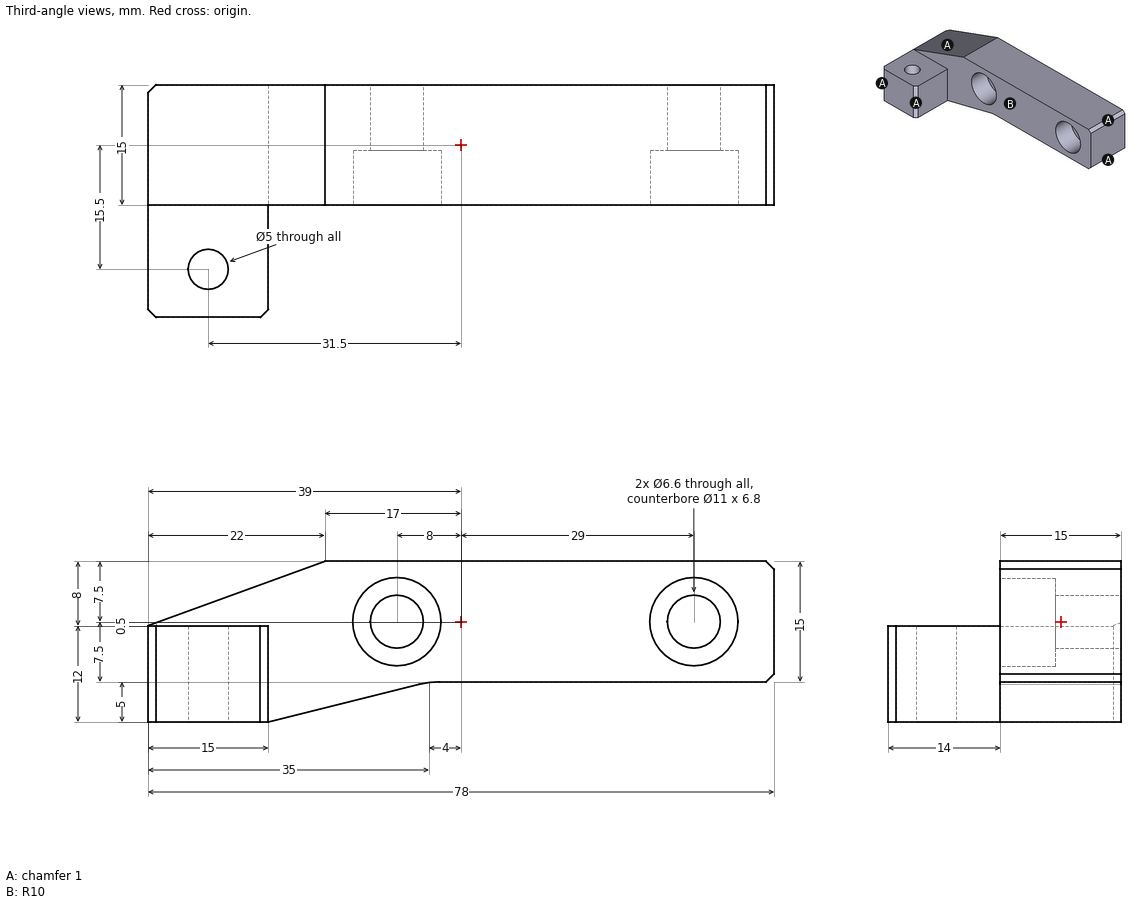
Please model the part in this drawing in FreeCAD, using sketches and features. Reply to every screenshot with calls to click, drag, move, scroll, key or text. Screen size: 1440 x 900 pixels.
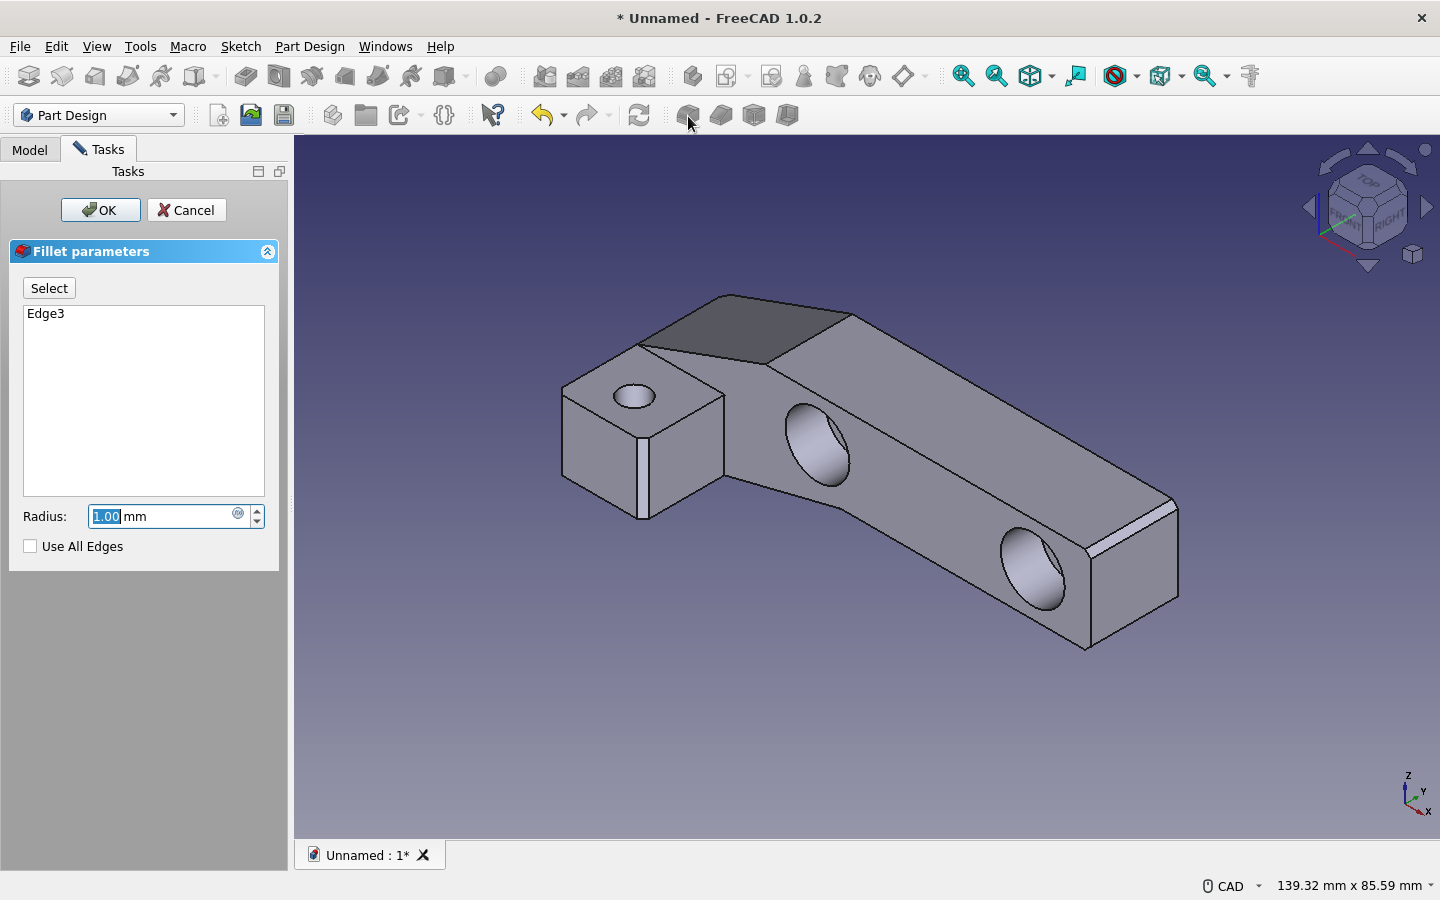
text(10)
key(Tab)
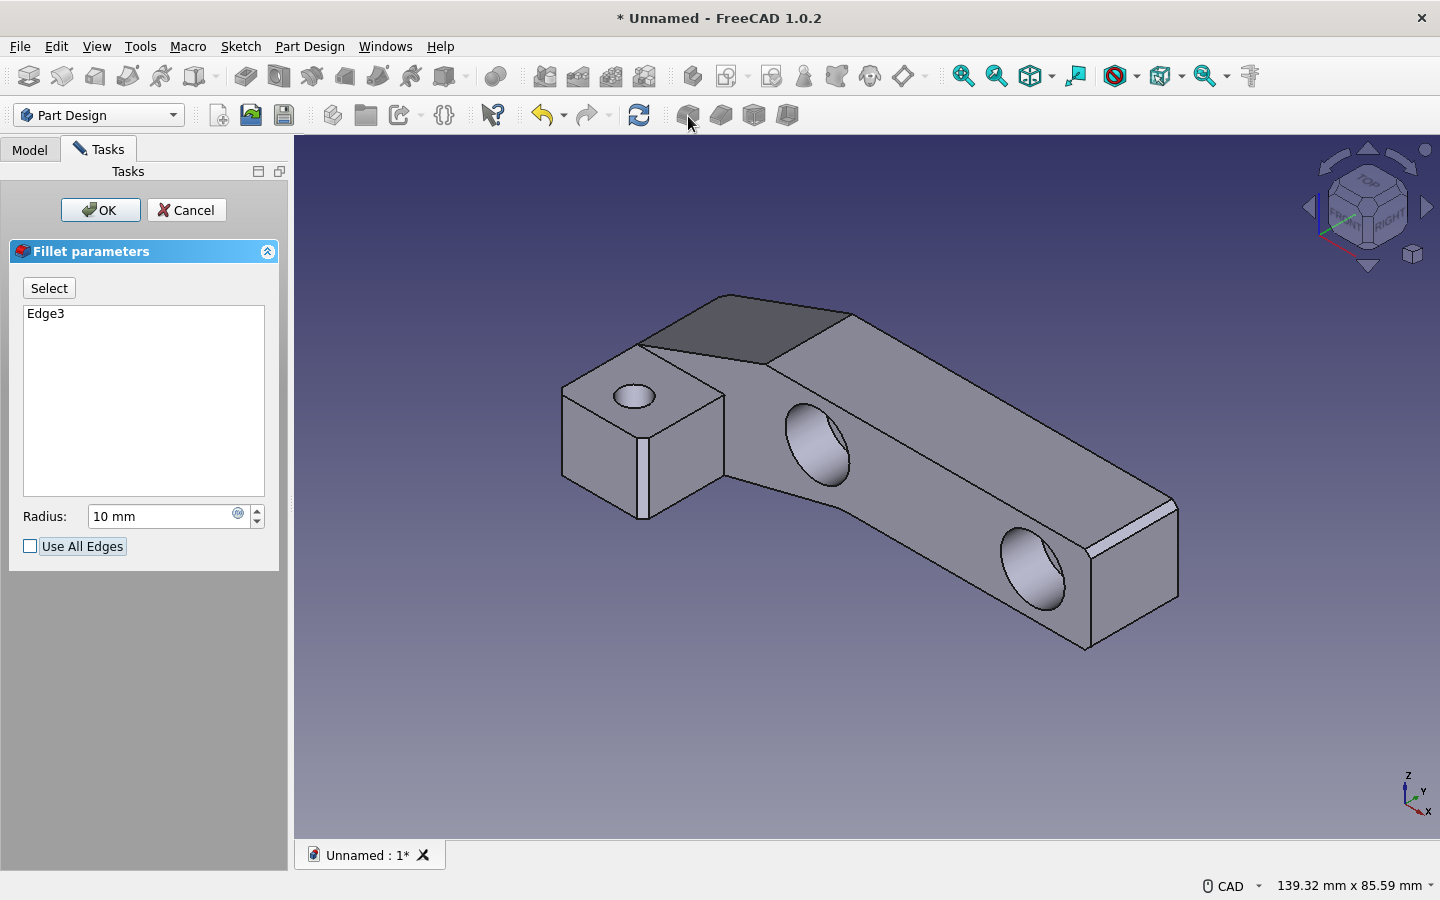
click(101, 210)